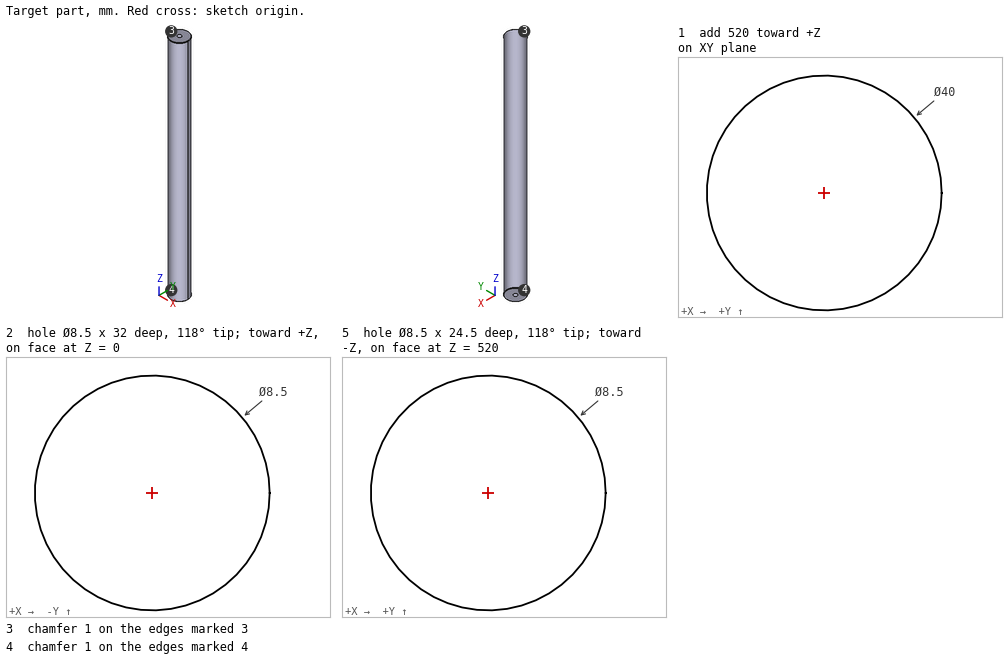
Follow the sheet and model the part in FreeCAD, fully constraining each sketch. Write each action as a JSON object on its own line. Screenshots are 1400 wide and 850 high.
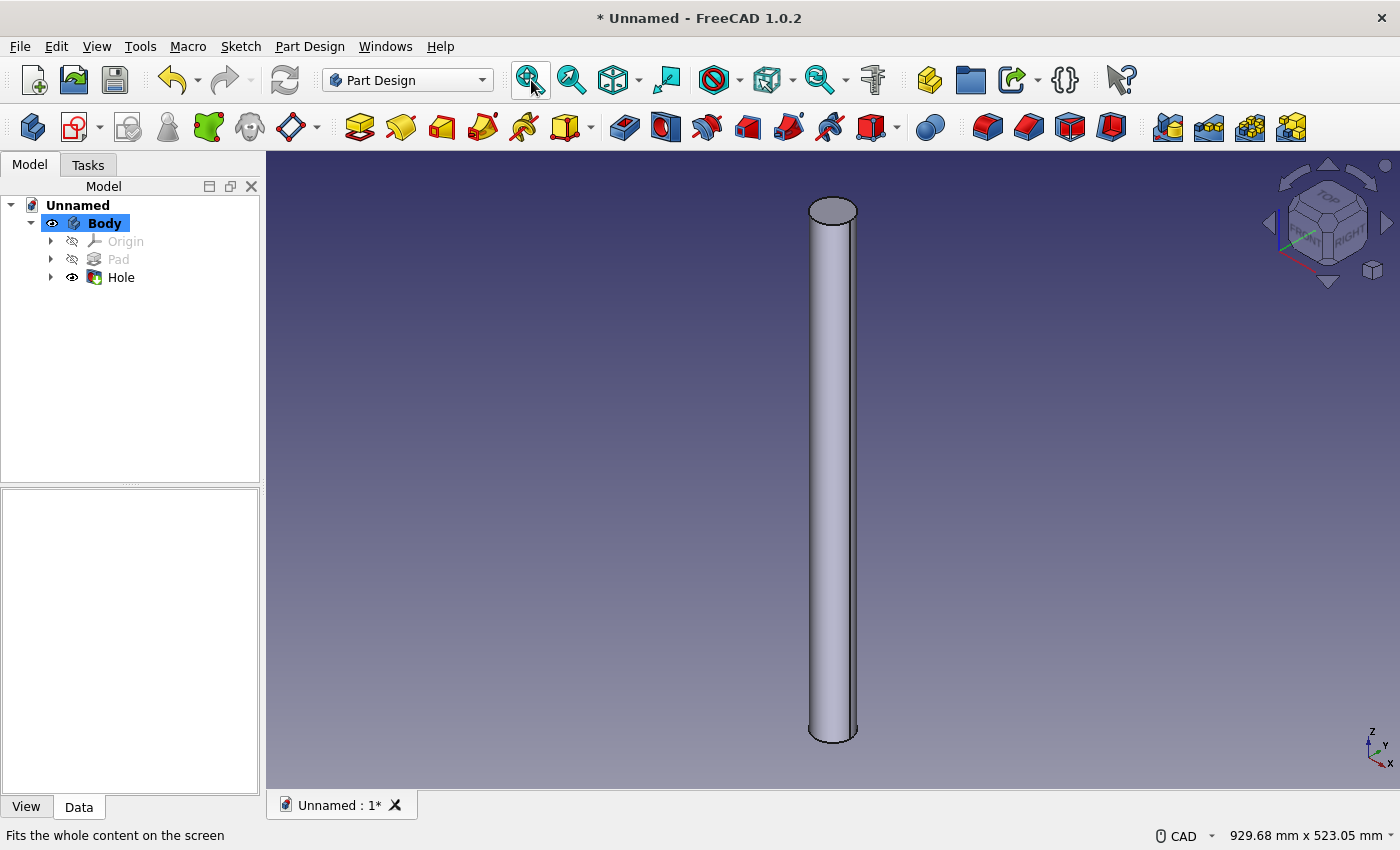
{"action": "left_click", "coordinate": [809, 208]}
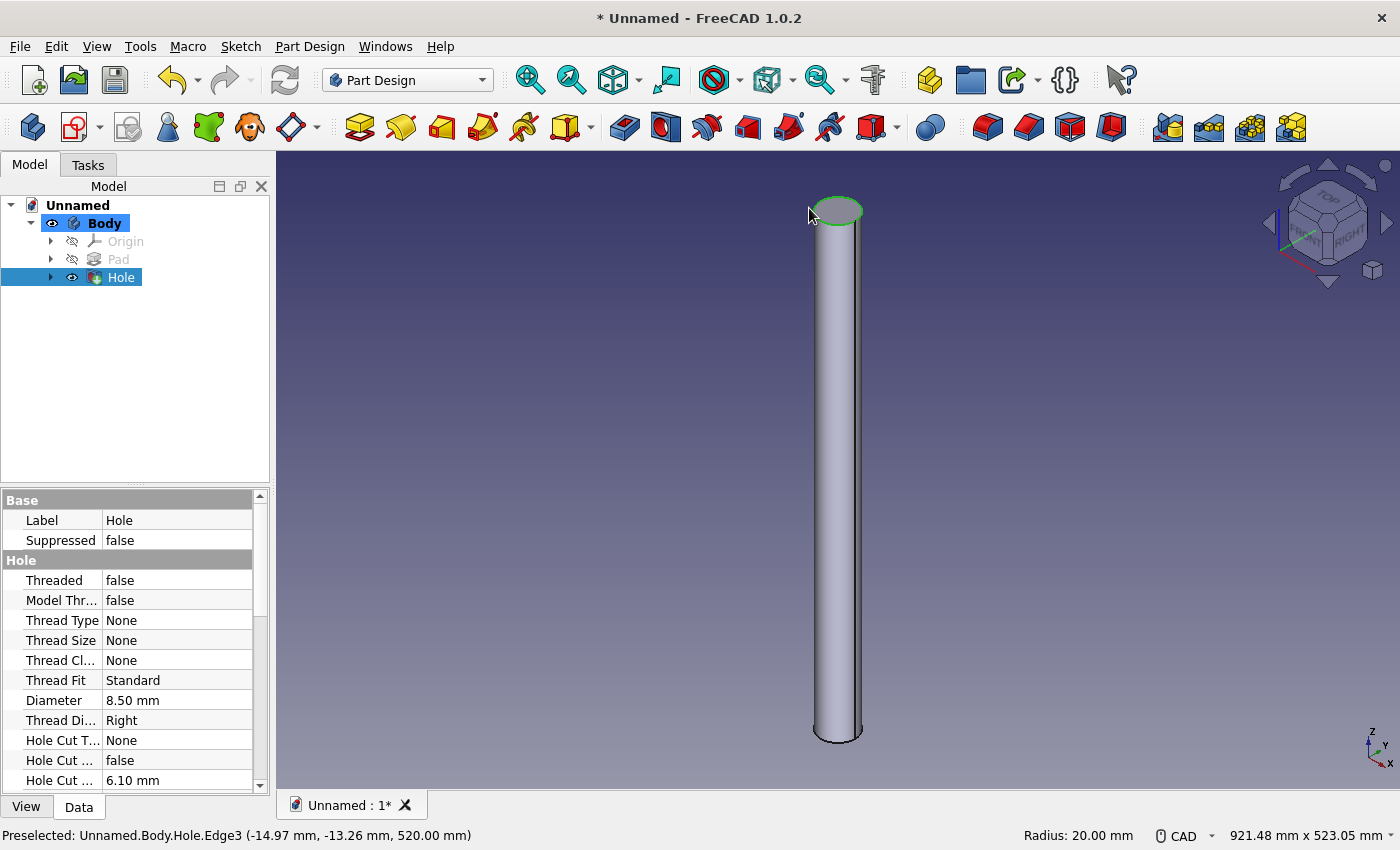
{"action": "left_click", "coordinate": [1029, 128]}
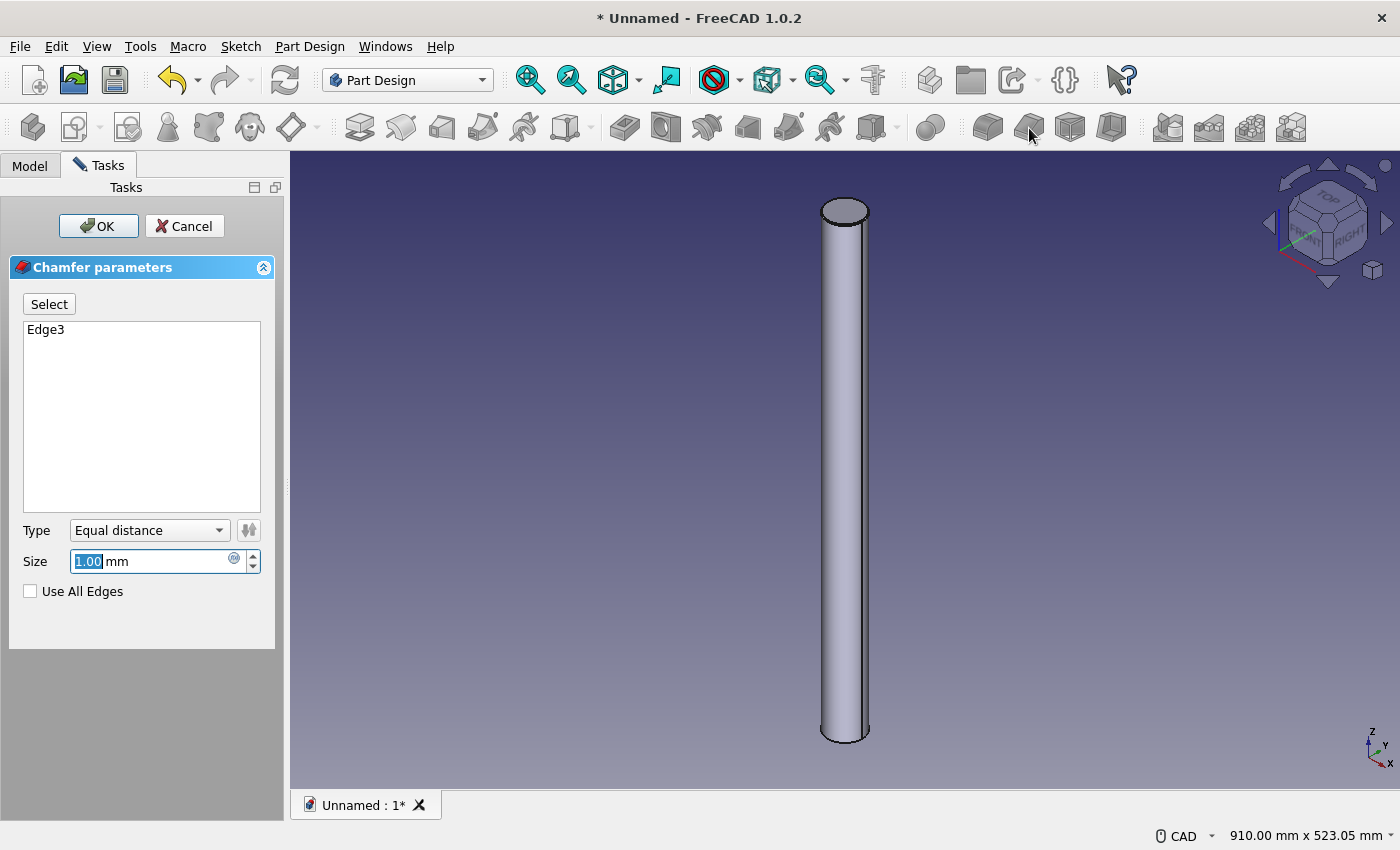
{"action": "type", "text": "1"}
{"action": "key", "text": "Tab"}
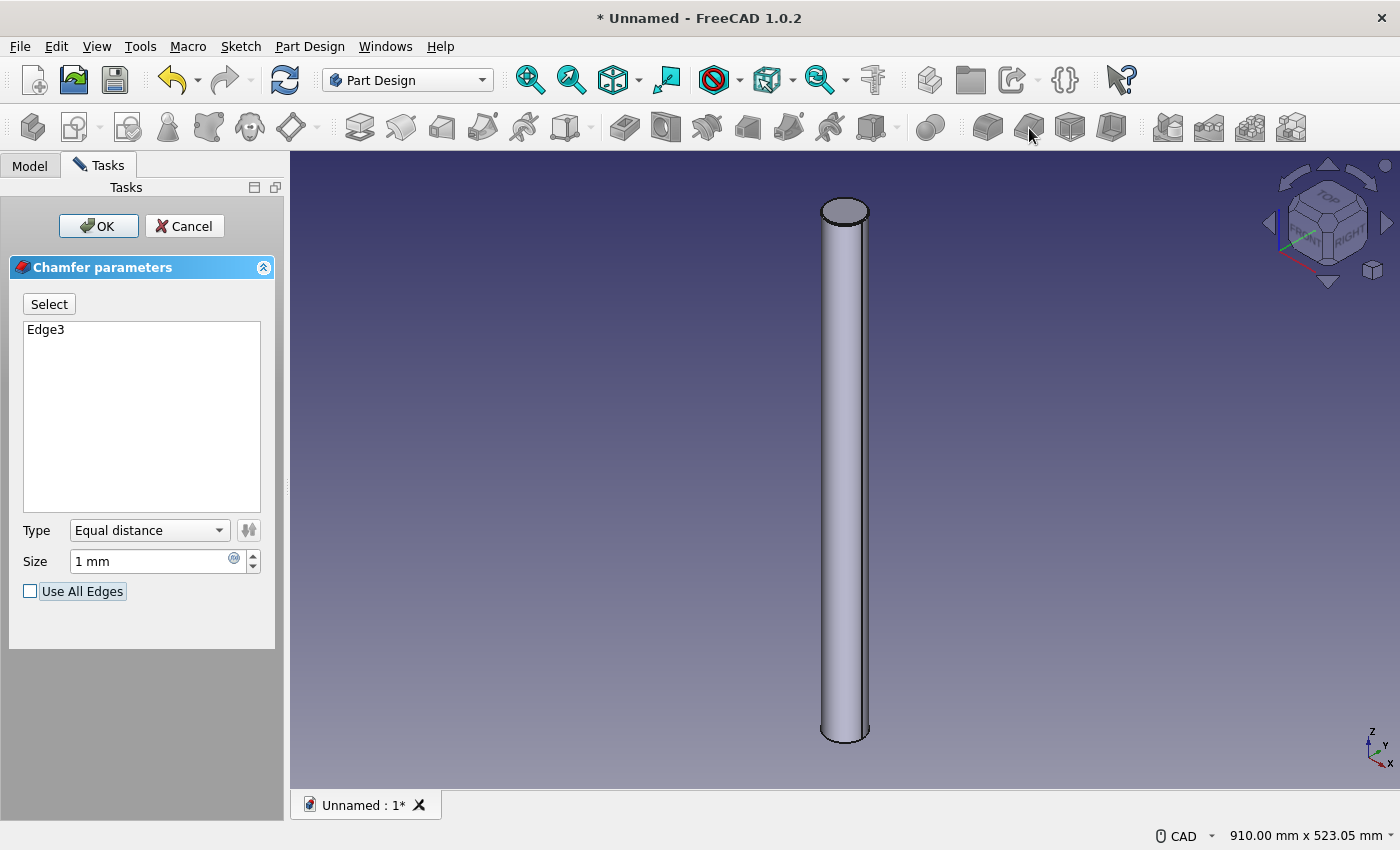
{"action": "left_click", "coordinate": [99, 226]}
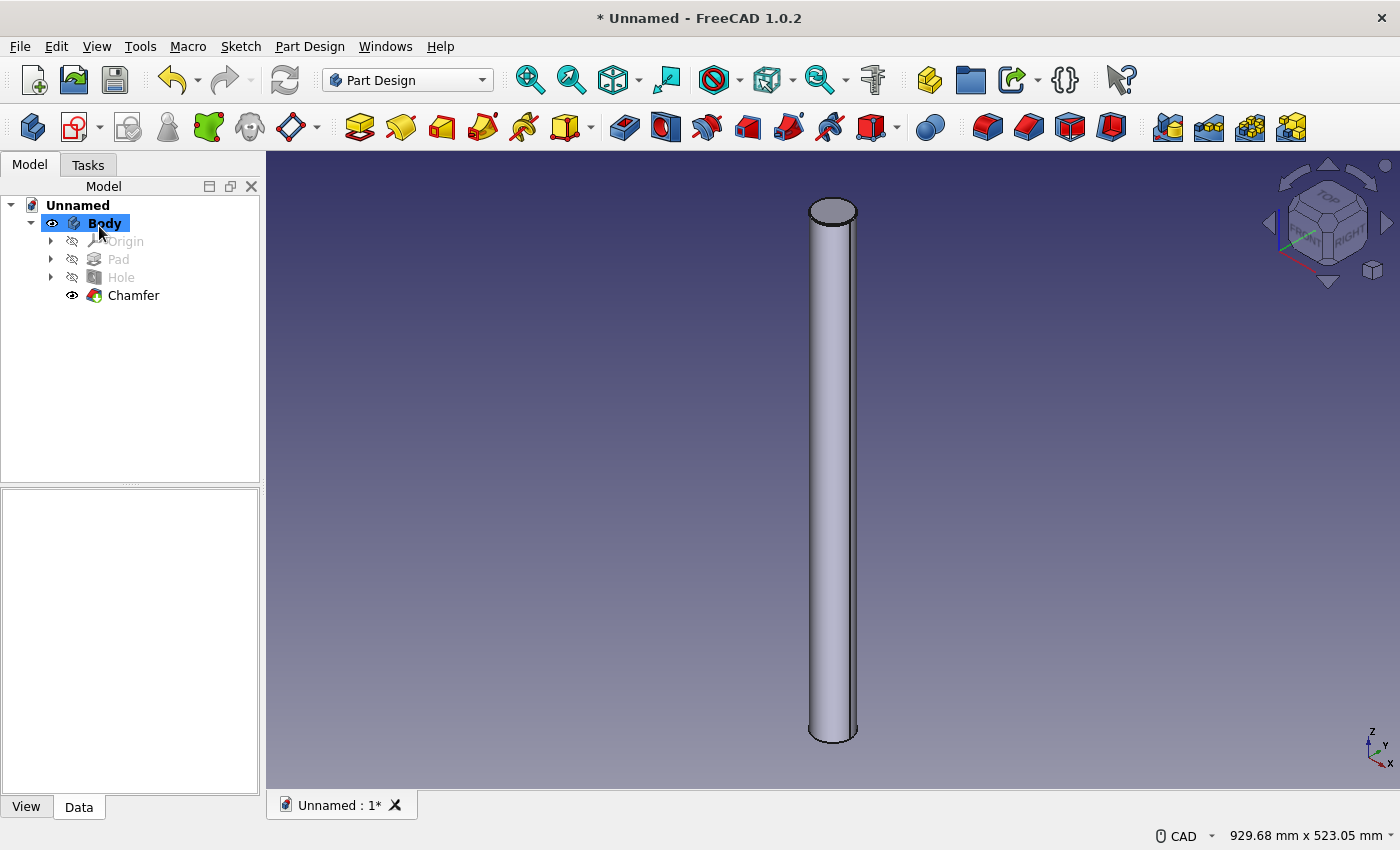
{"action": "left_click", "coordinate": [811, 734]}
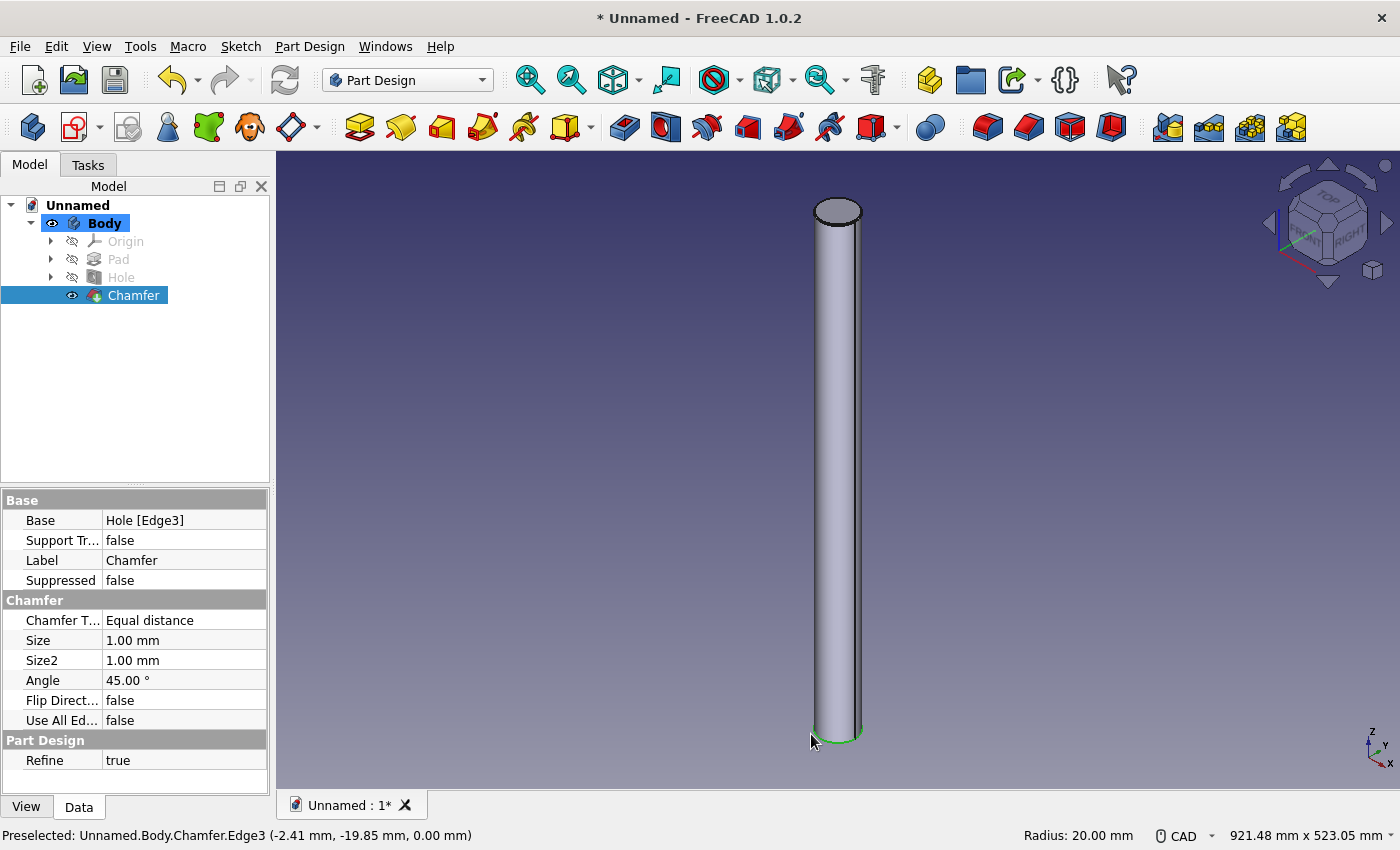
{"action": "left_click", "coordinate": [1029, 128]}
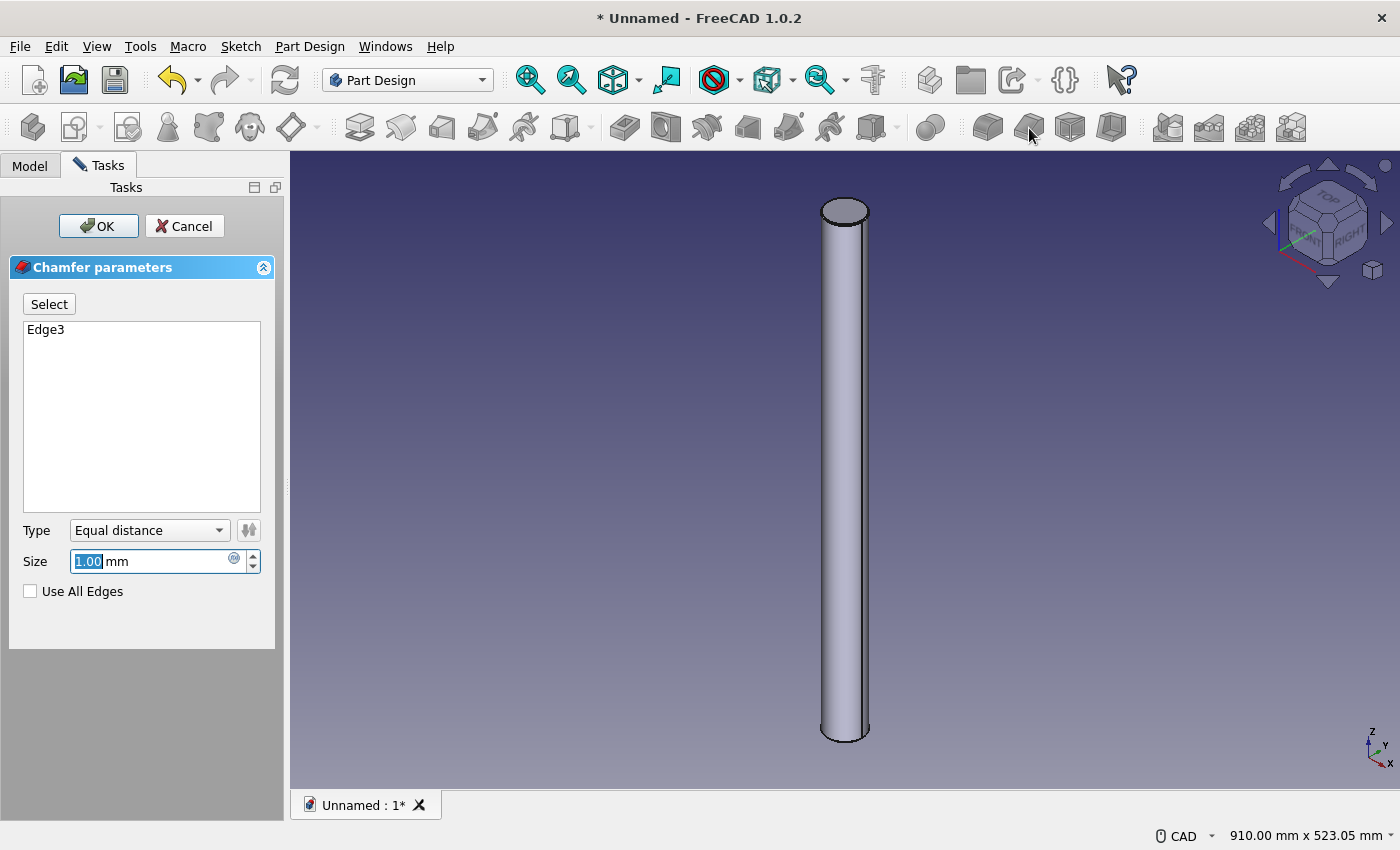
{"action": "type", "text": "1"}
{"action": "key", "text": "Tab"}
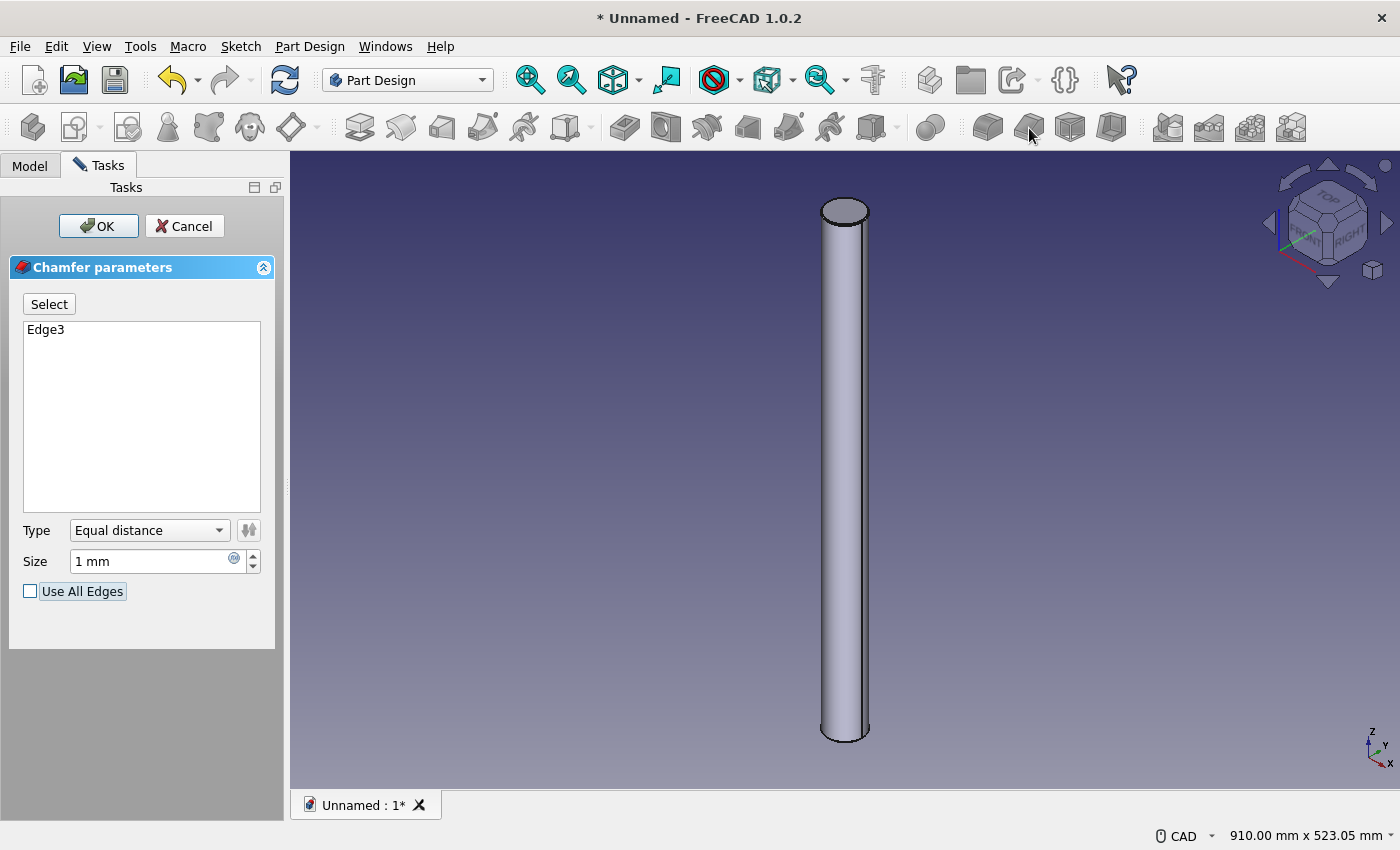
{"action": "left_click", "coordinate": [99, 226]}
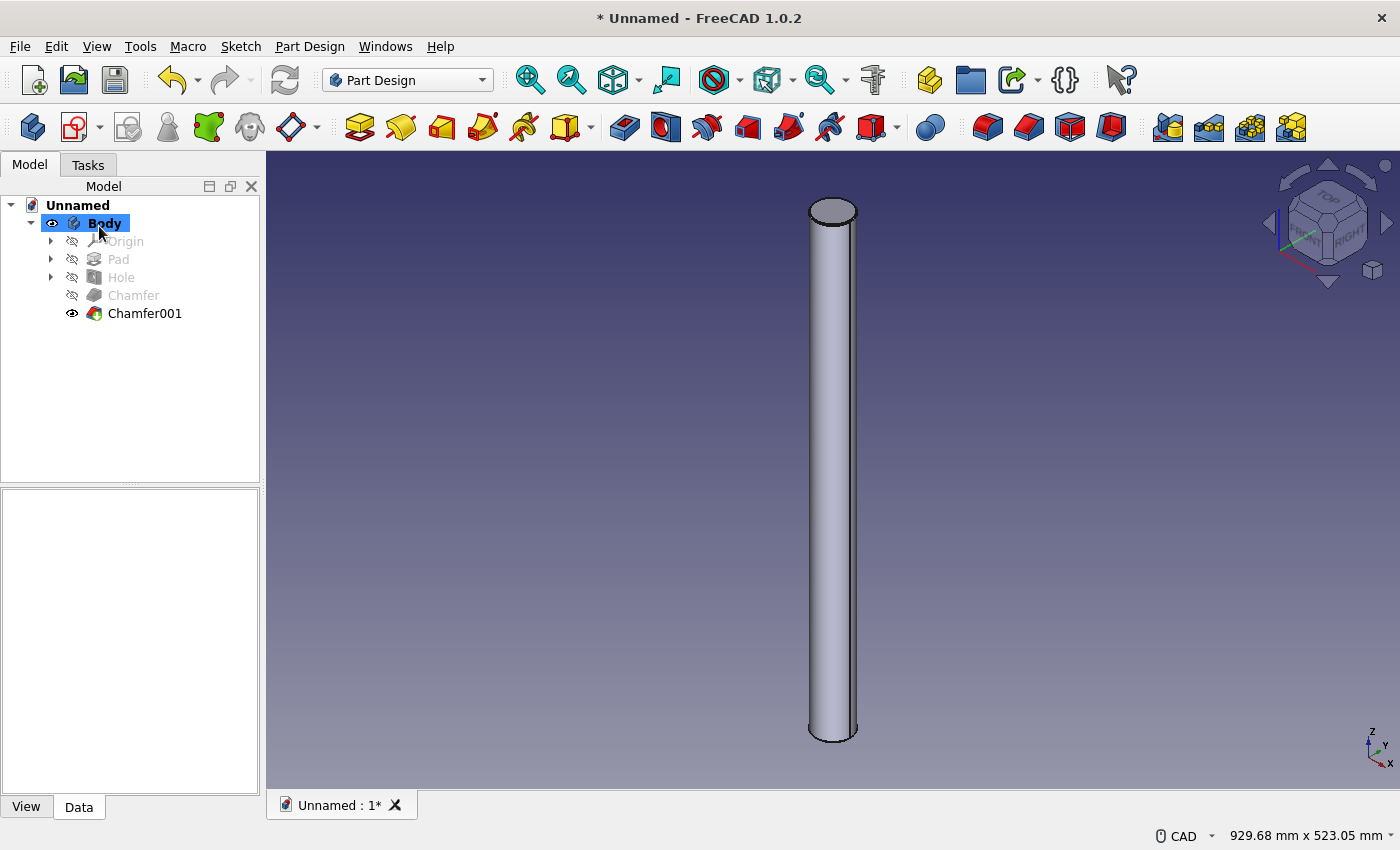
{"action": "left_click", "coordinate": [833, 210]}